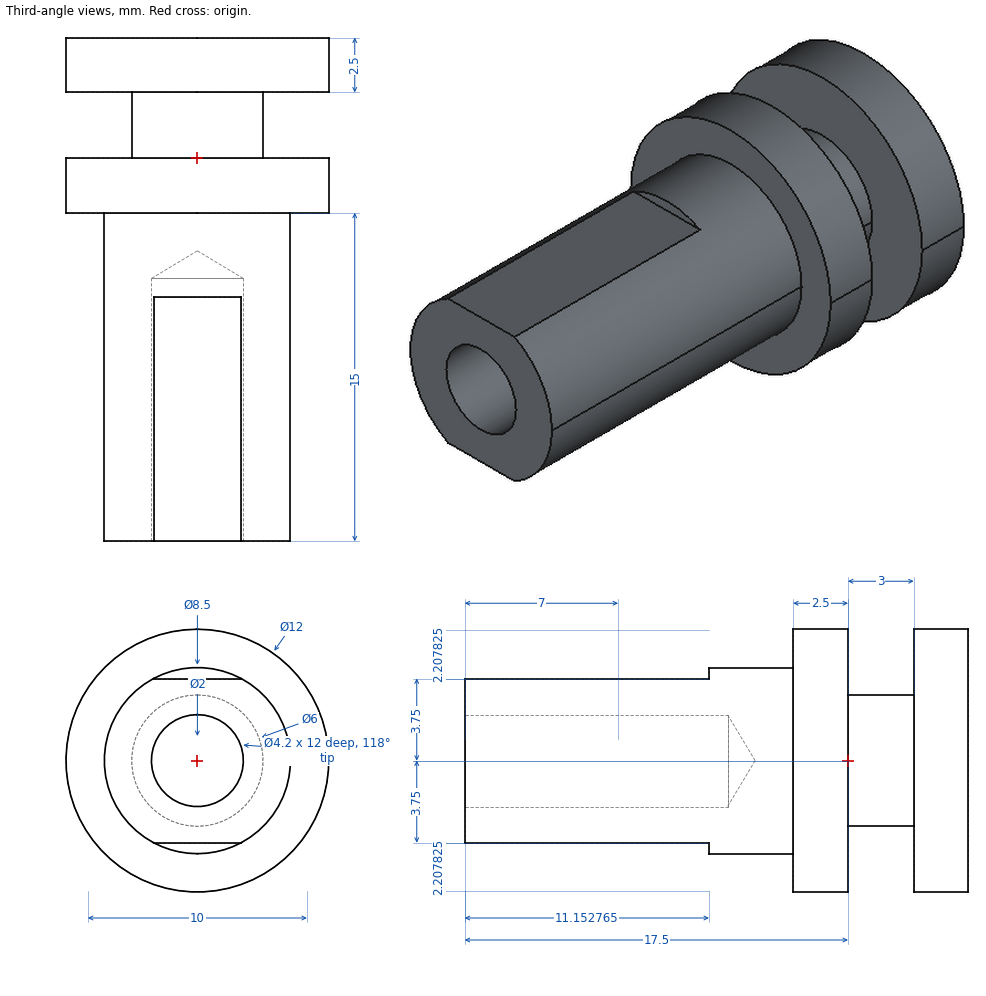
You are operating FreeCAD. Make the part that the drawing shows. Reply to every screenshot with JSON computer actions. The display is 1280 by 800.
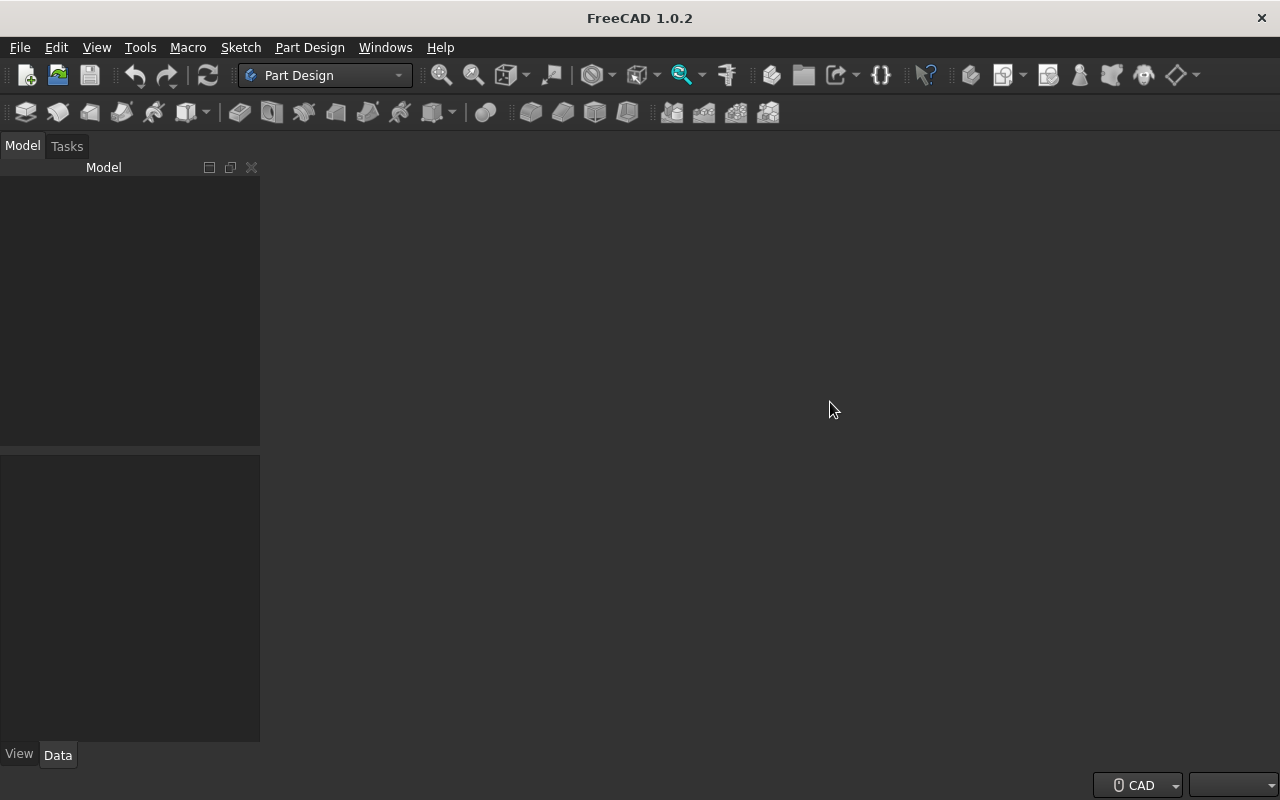
{"action": "left_click", "coordinate": [26, 76]}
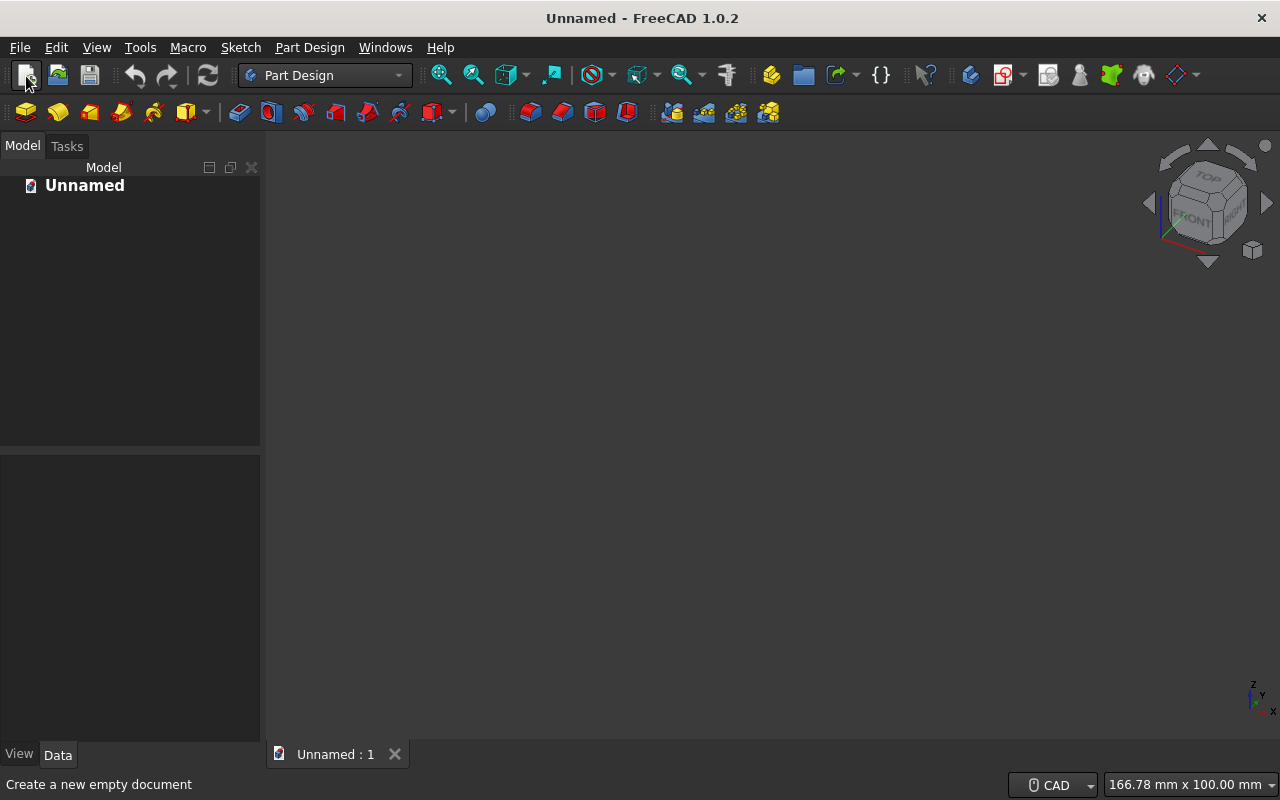
{"action": "left_click", "coordinate": [1004, 76]}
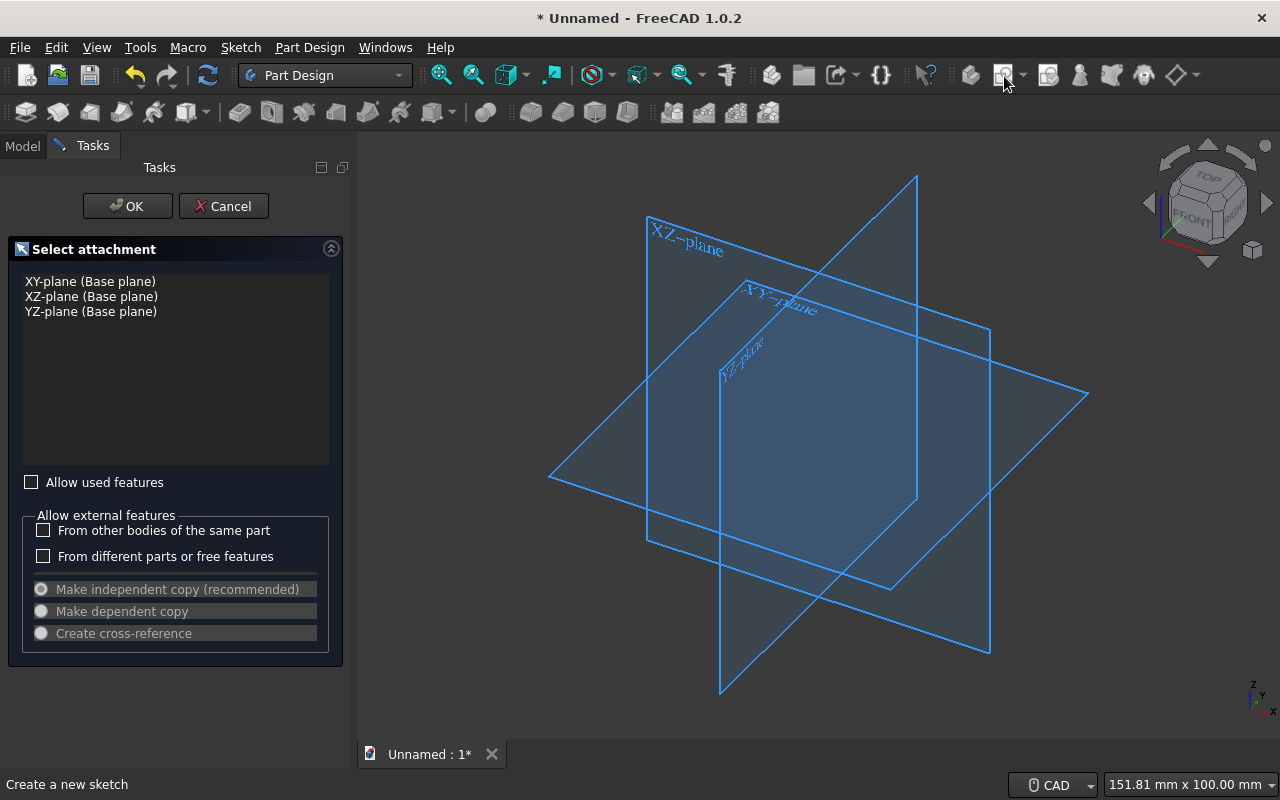
{"action": "left_click", "coordinate": [82, 296]}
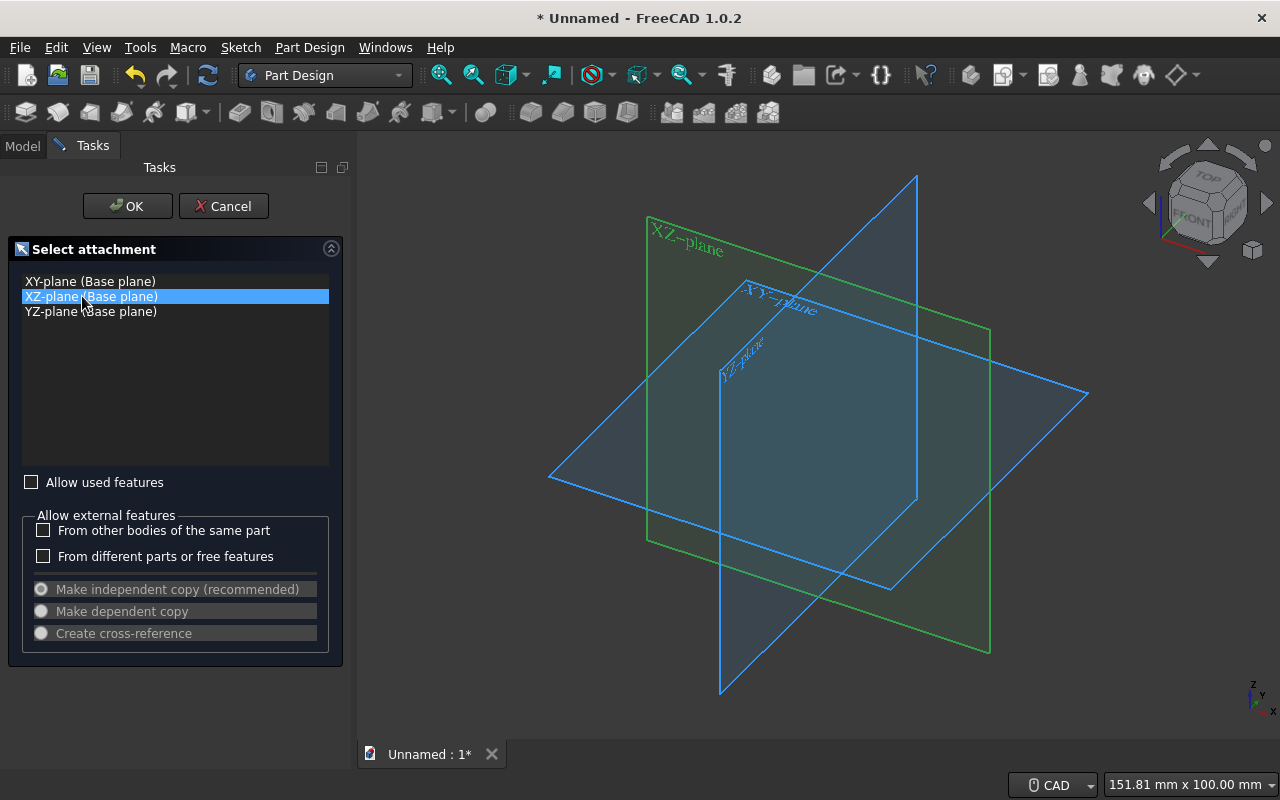
{"action": "left_click", "coordinate": [128, 206]}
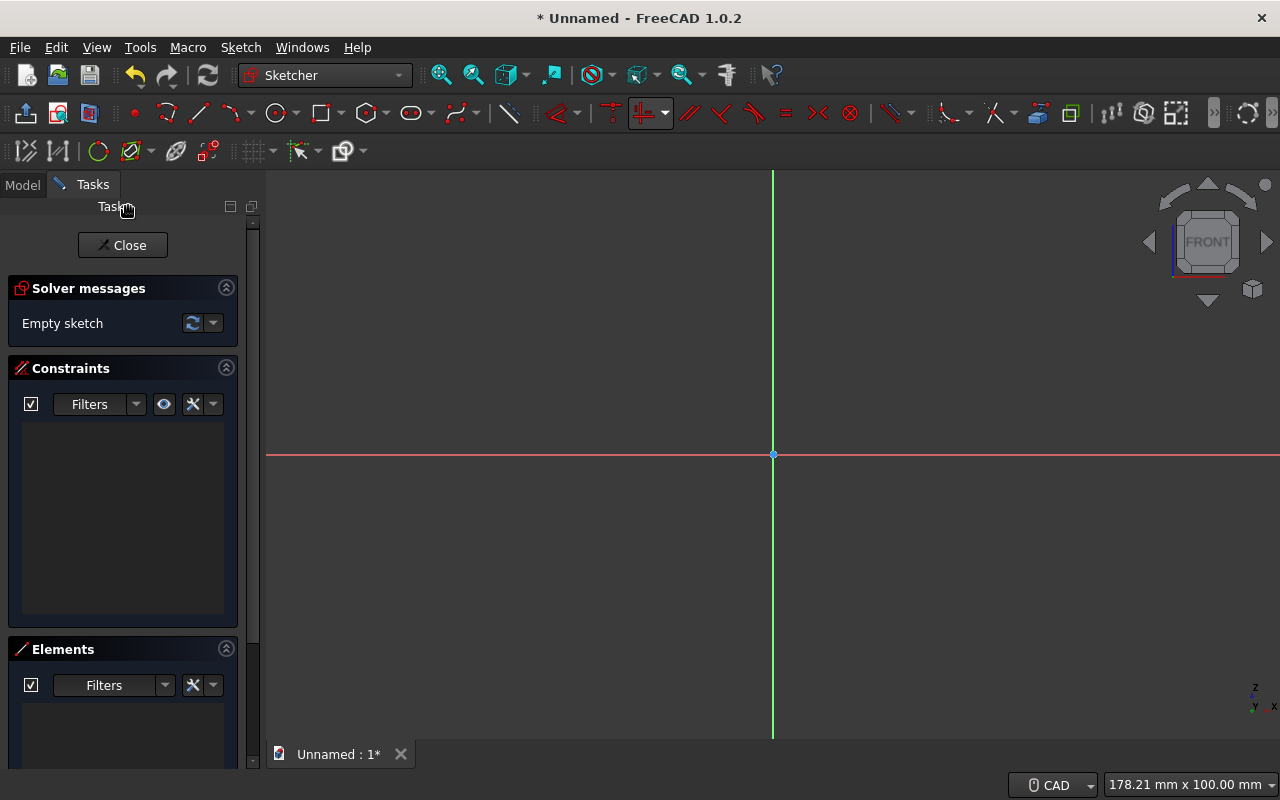
{"action": "scroll", "coordinate": [780, 455], "scroll_direction": "up", "scroll_amount": 12}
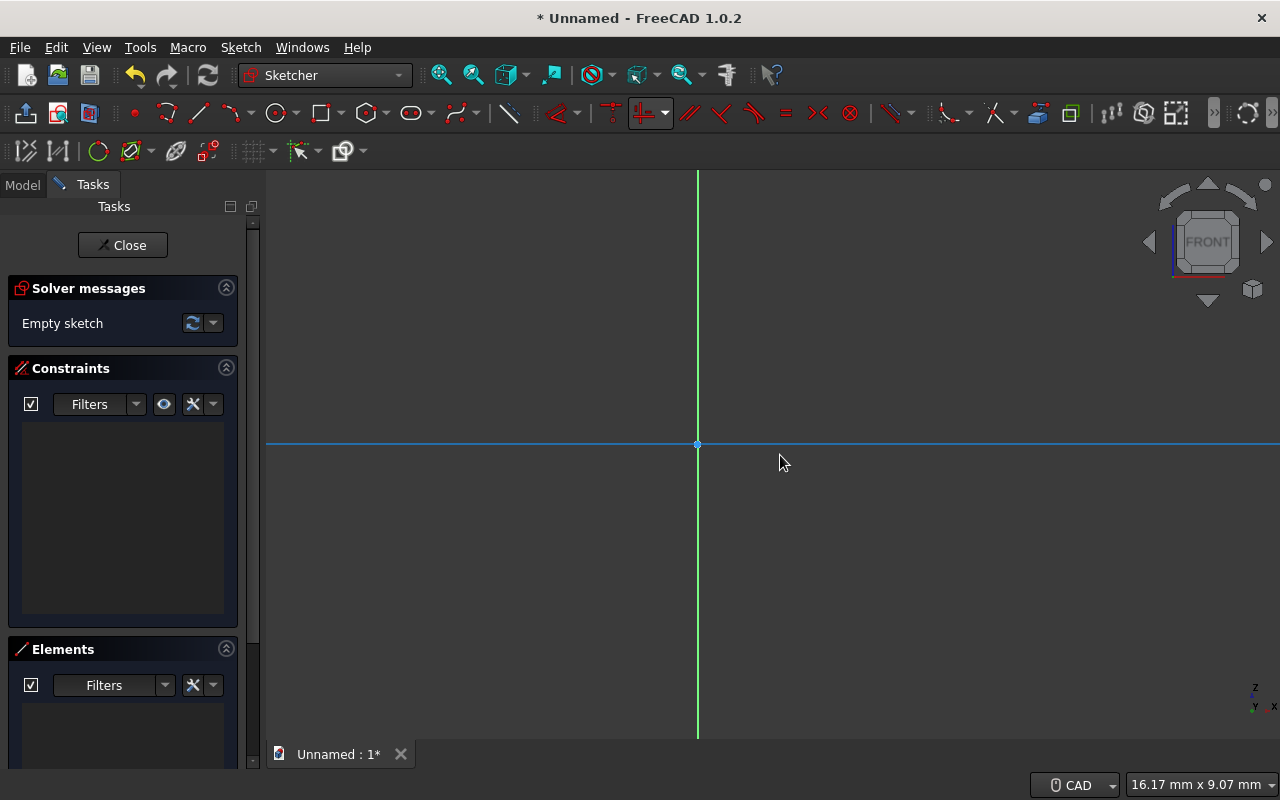
{"action": "key", "text": "g c"}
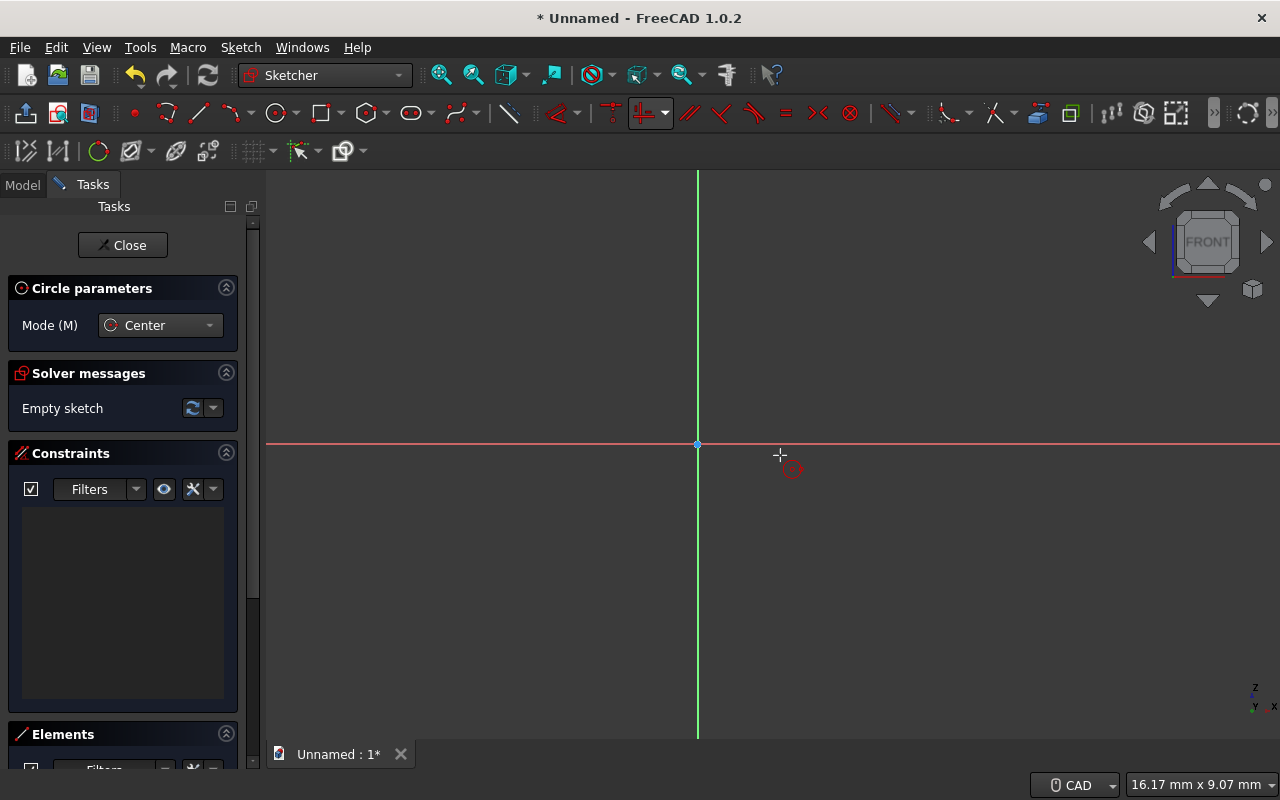
{"action": "left_click", "coordinate": [698, 444]}
{"action": "mouse_move", "coordinate": [831, 311]}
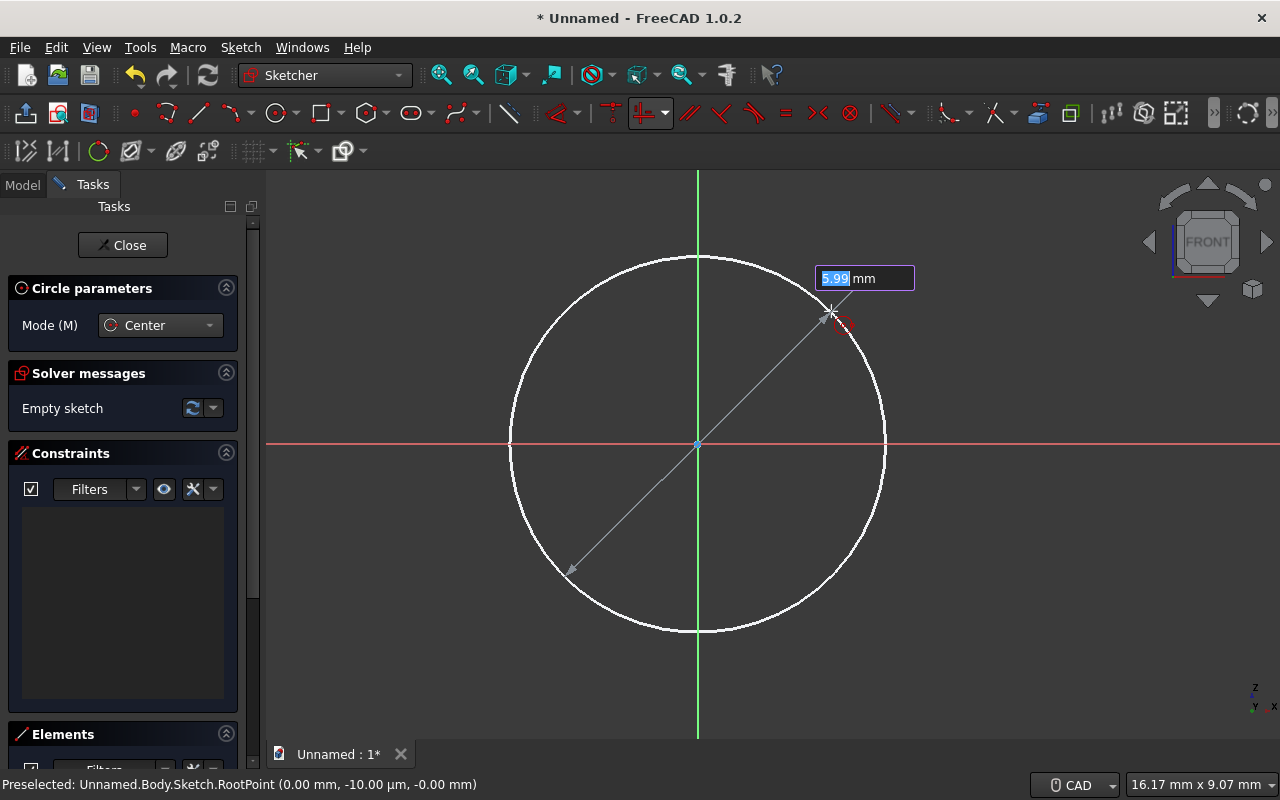
{"action": "type", "text": "6"}
{"action": "key", "text": "Return"}
{"action": "key", "text": "Escape"}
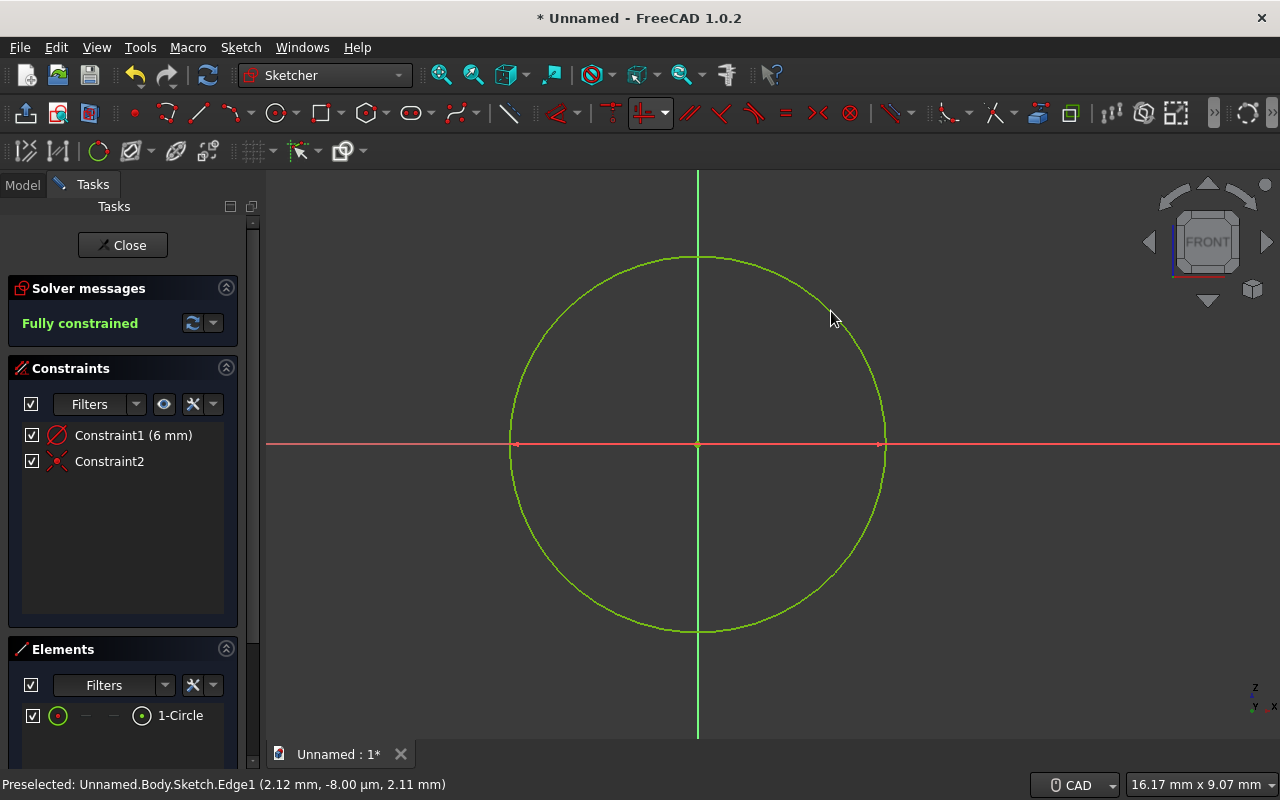
{"action": "left_click", "coordinate": [123, 245]}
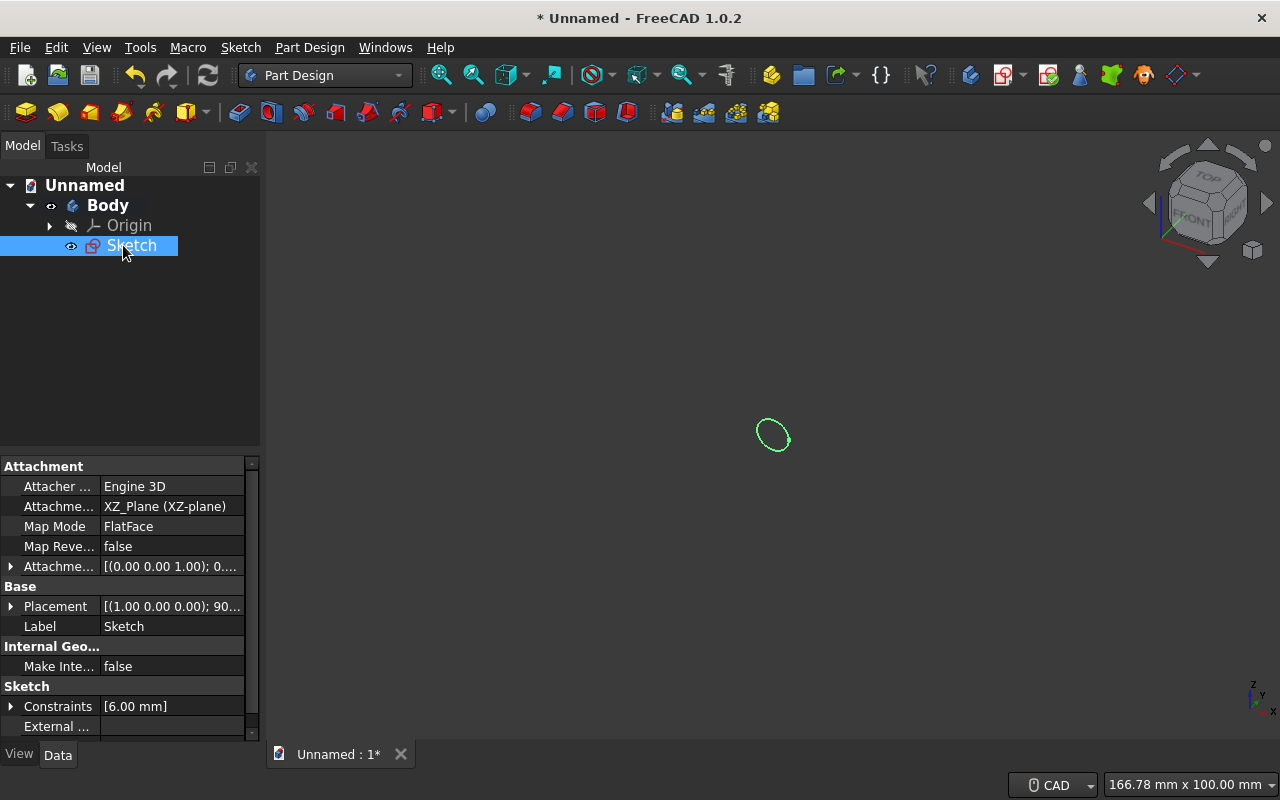
{"action": "left_click", "coordinate": [26, 112]}